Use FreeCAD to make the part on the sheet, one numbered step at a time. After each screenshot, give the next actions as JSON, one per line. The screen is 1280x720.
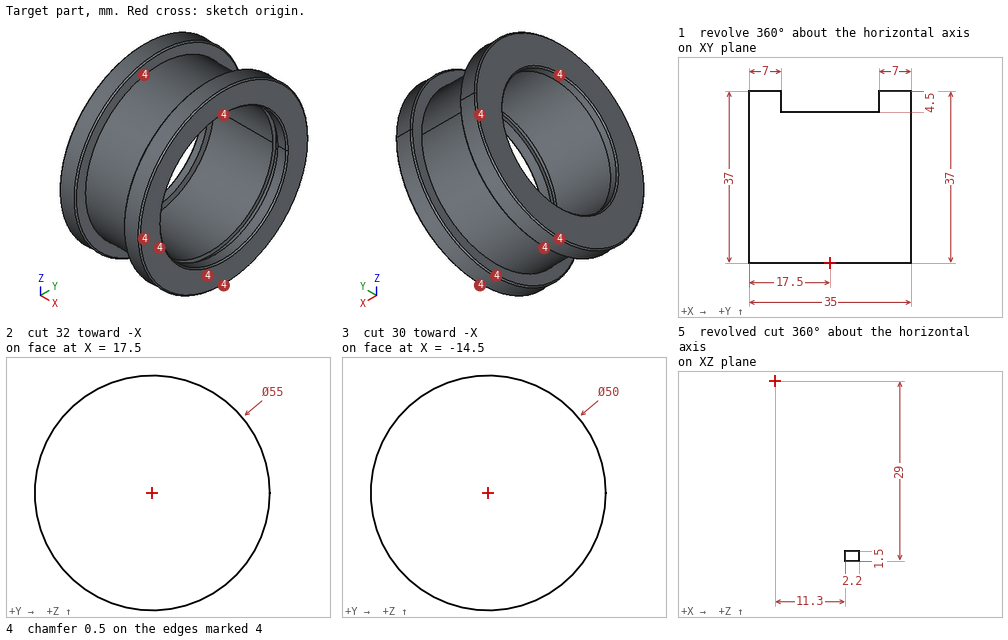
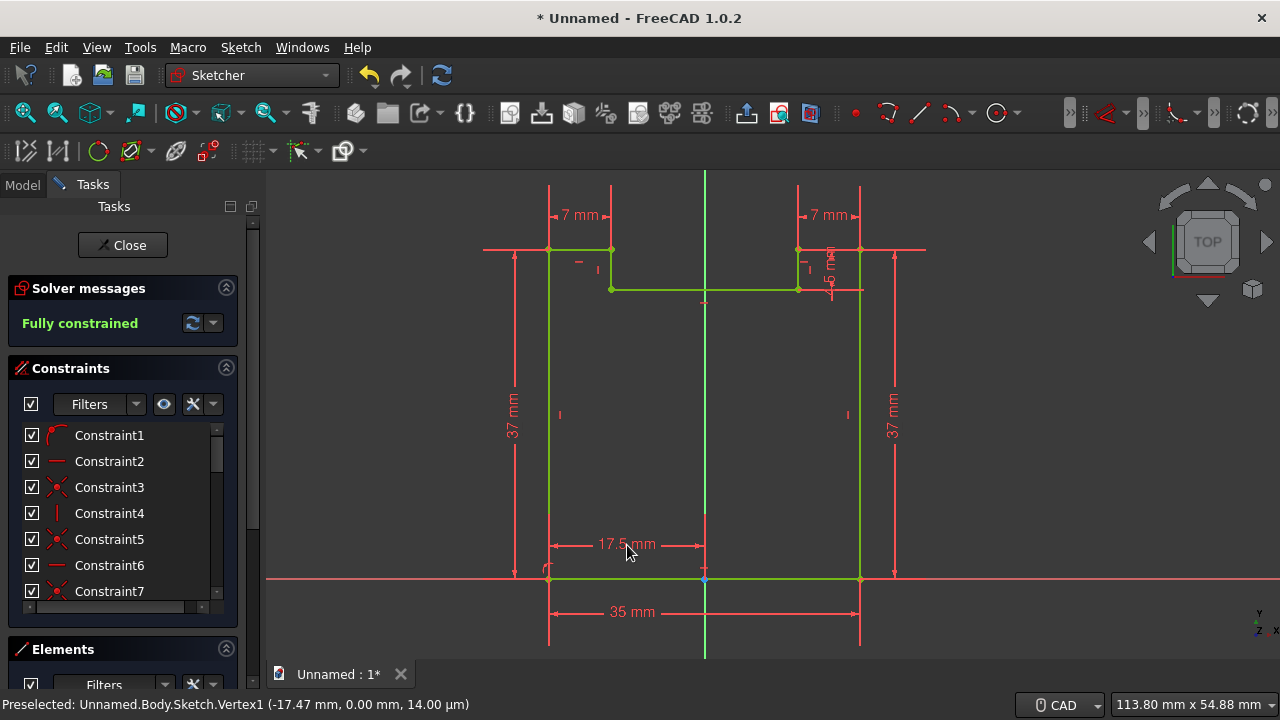
{"action": "left_click", "coordinate": [123, 245]}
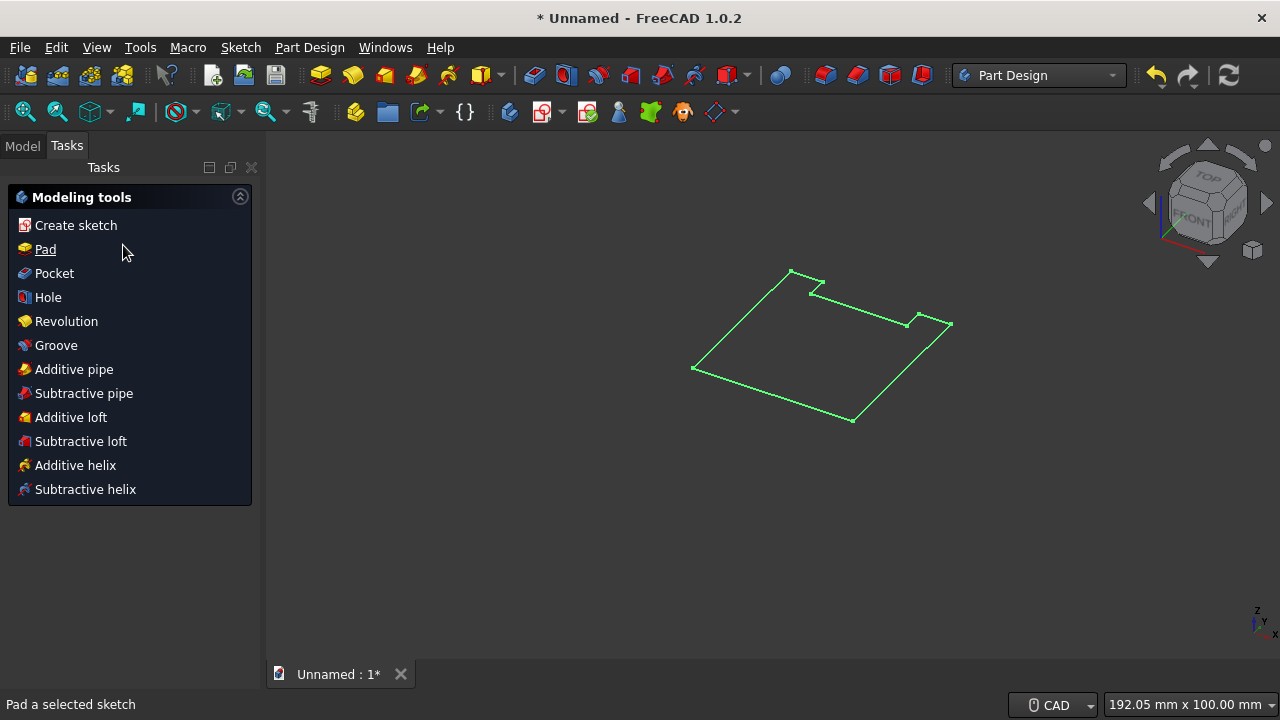
{"action": "left_click", "coordinate": [354, 76]}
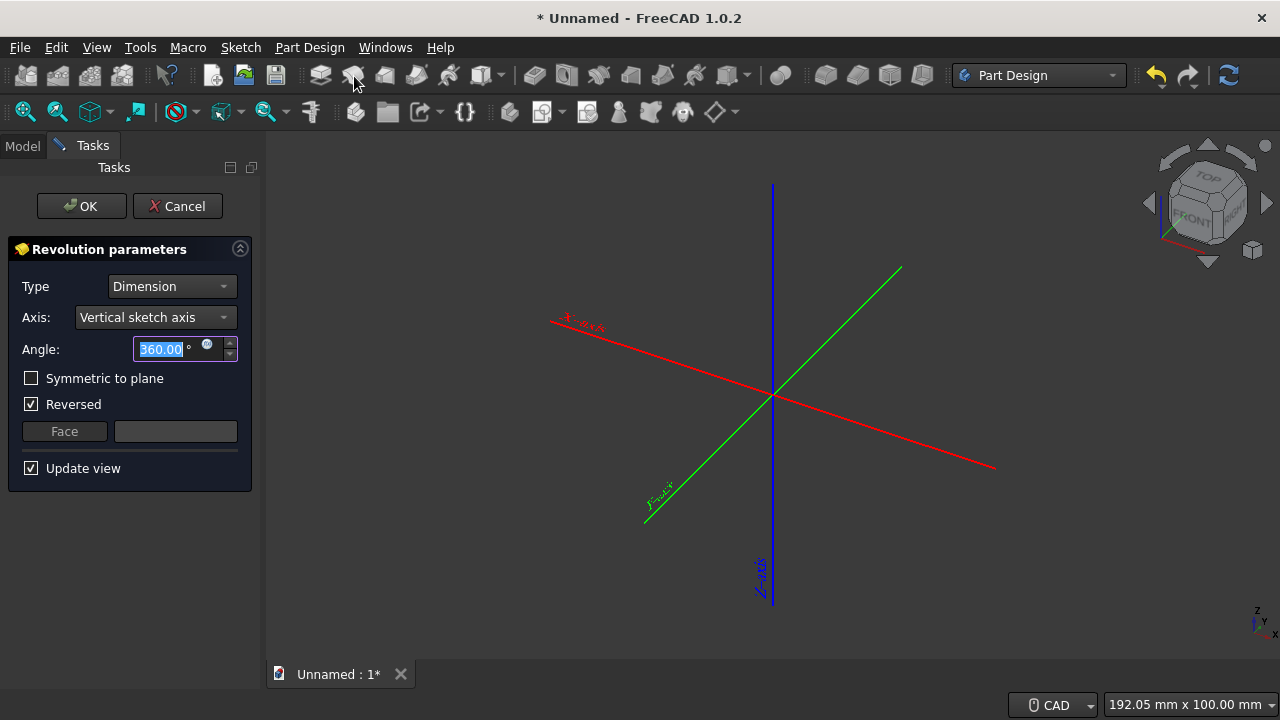
{"action": "left_click", "coordinate": [156, 318]}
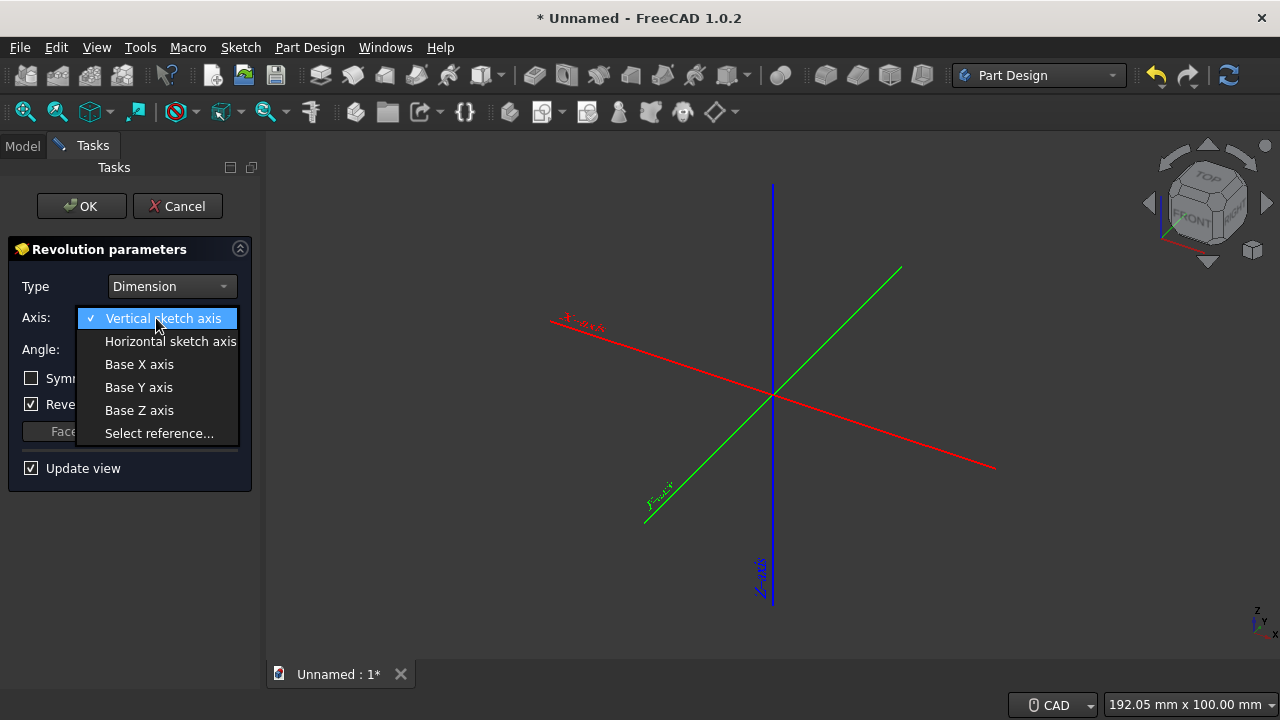
{"action": "left_click", "coordinate": [156, 342]}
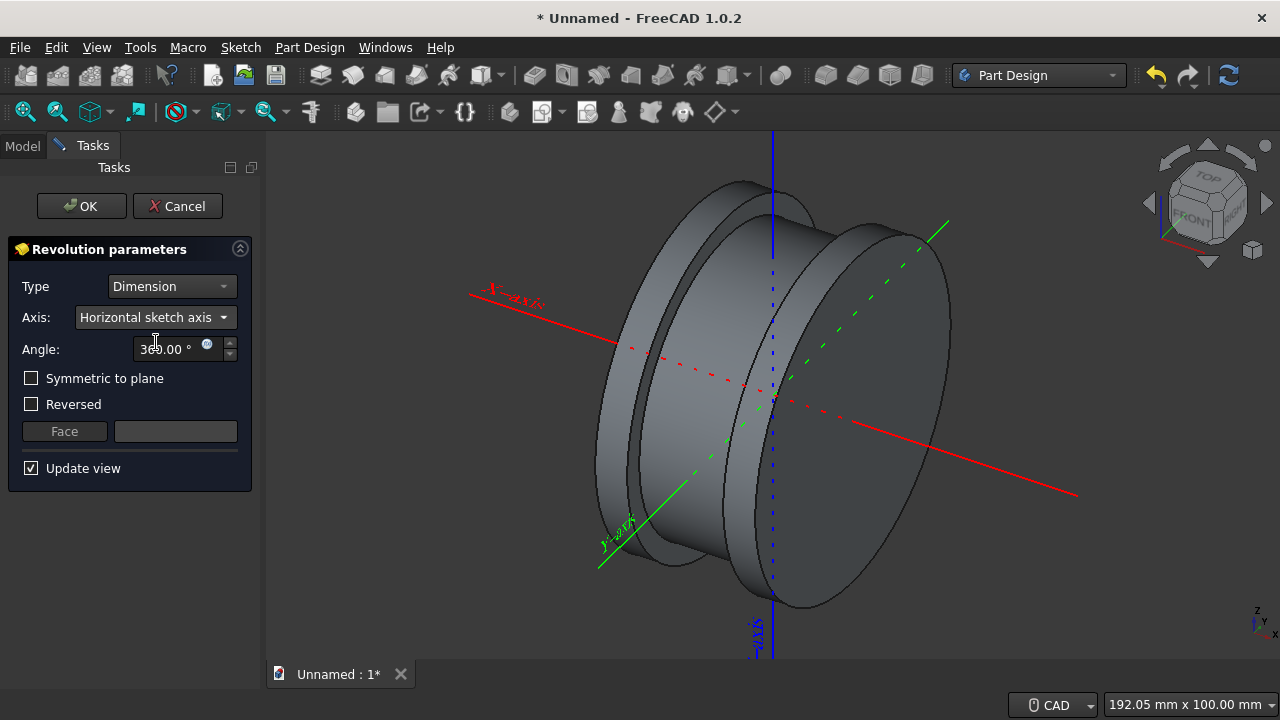
{"action": "left_click", "coordinate": [82, 206]}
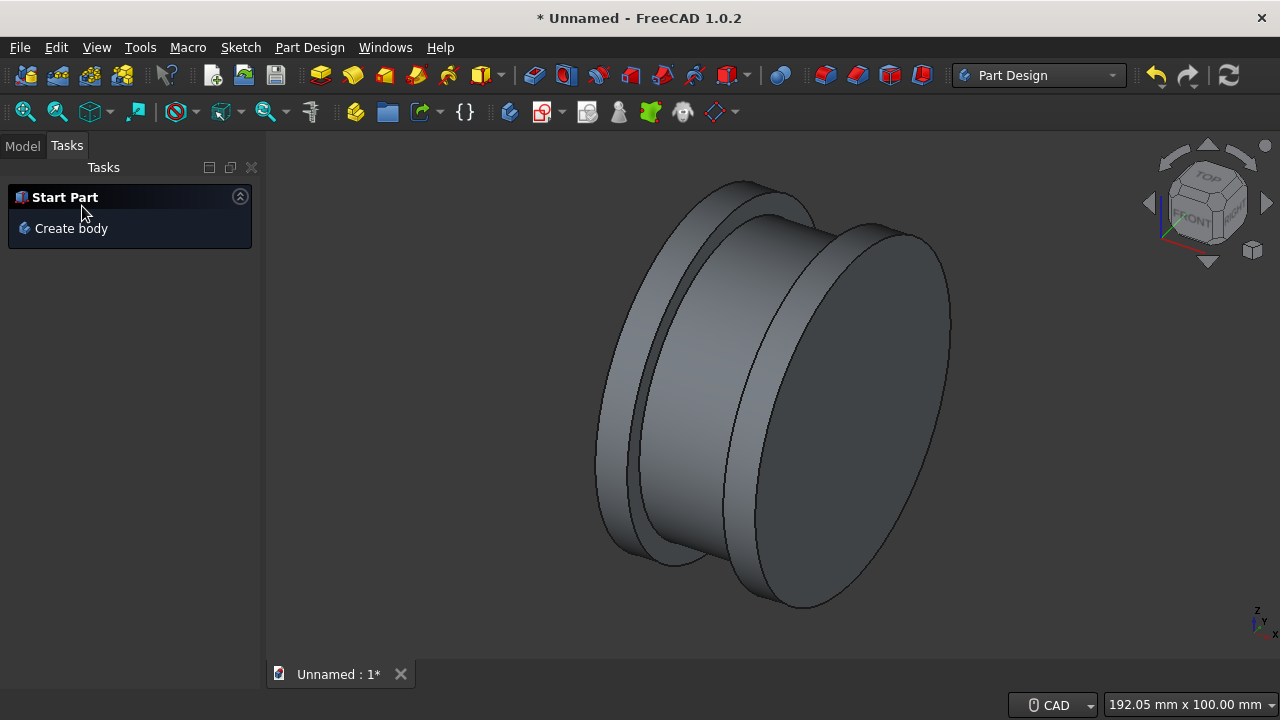
{"action": "key", "text": "v f"}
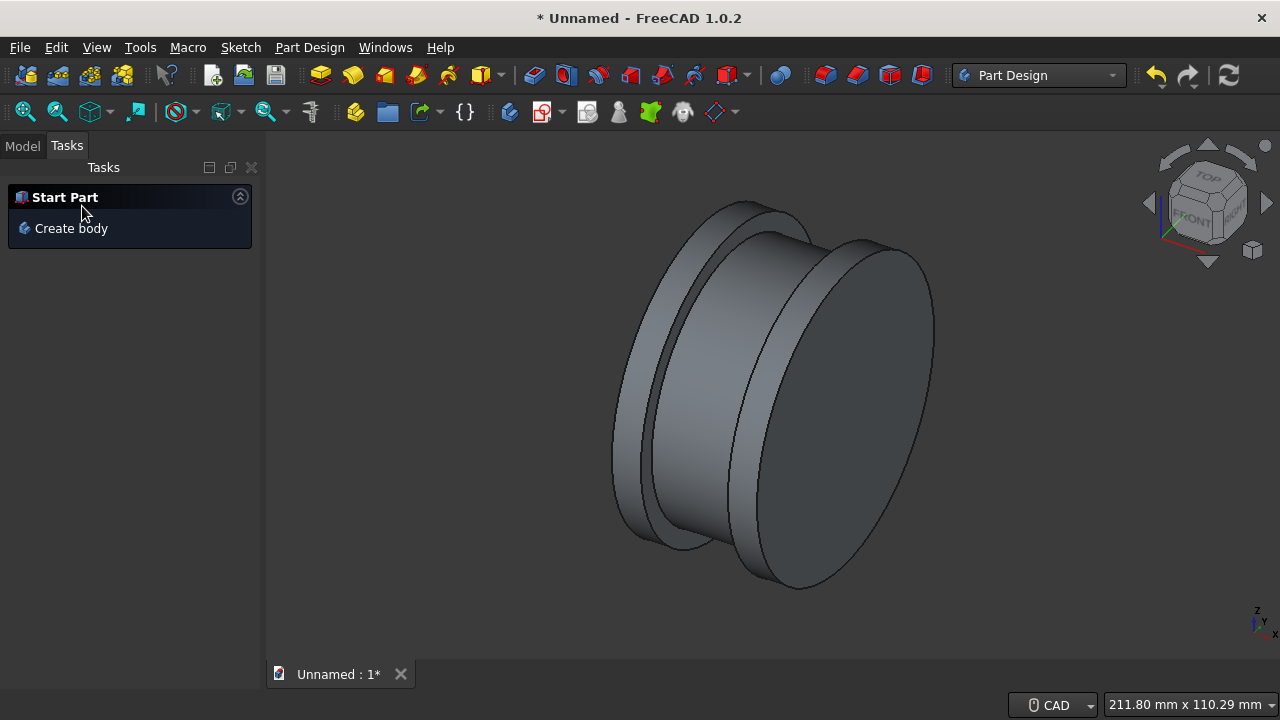
{"action": "left_click", "coordinate": [845, 418]}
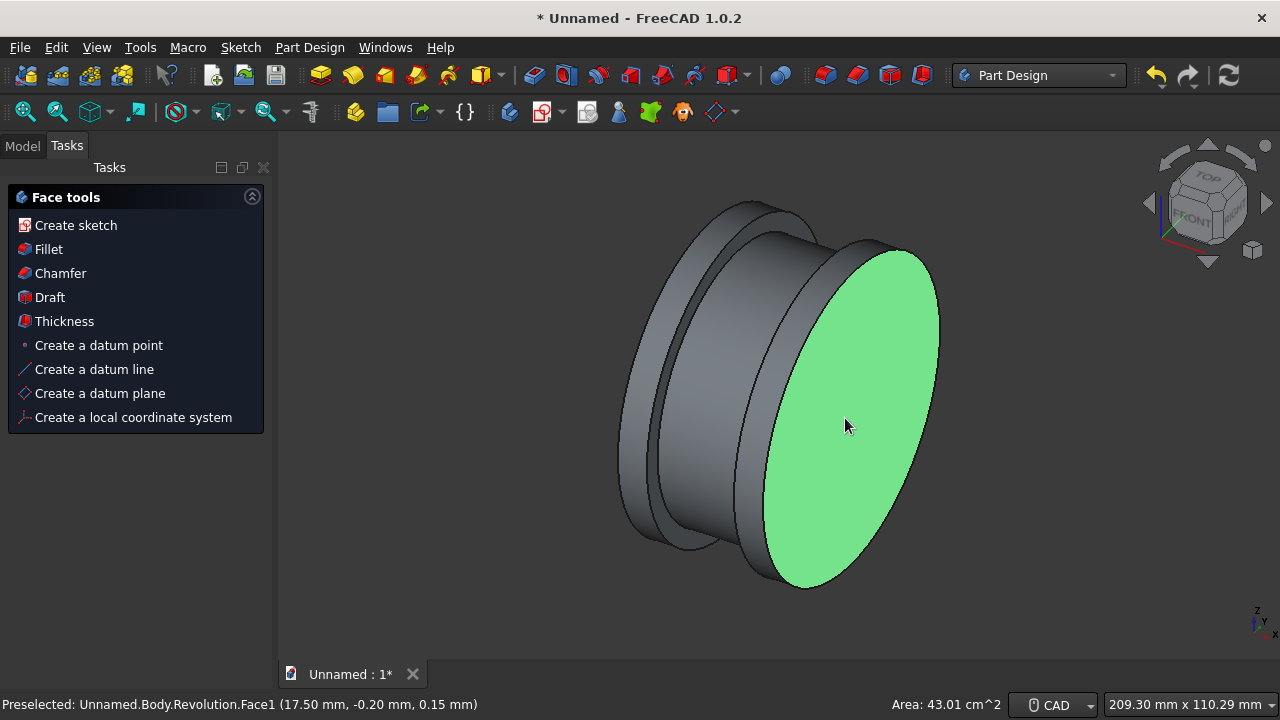
{"action": "left_click", "coordinate": [542, 112]}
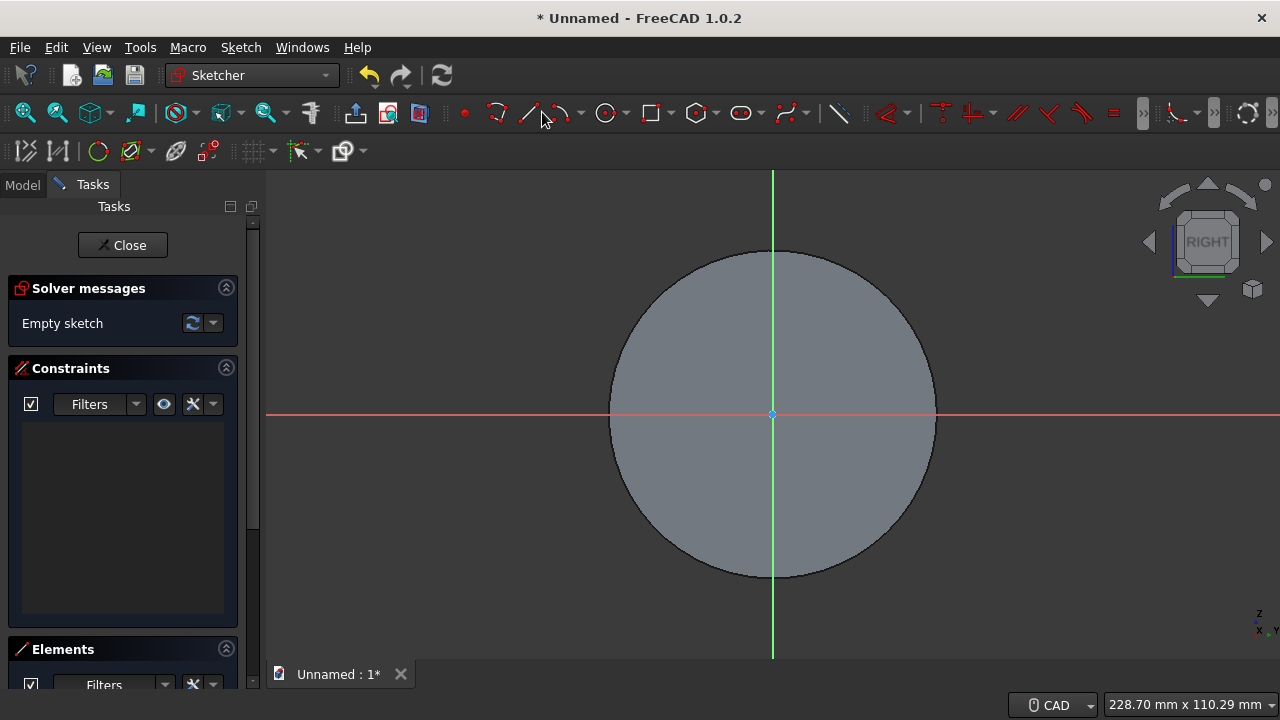
{"action": "left_click", "coordinate": [606, 114]}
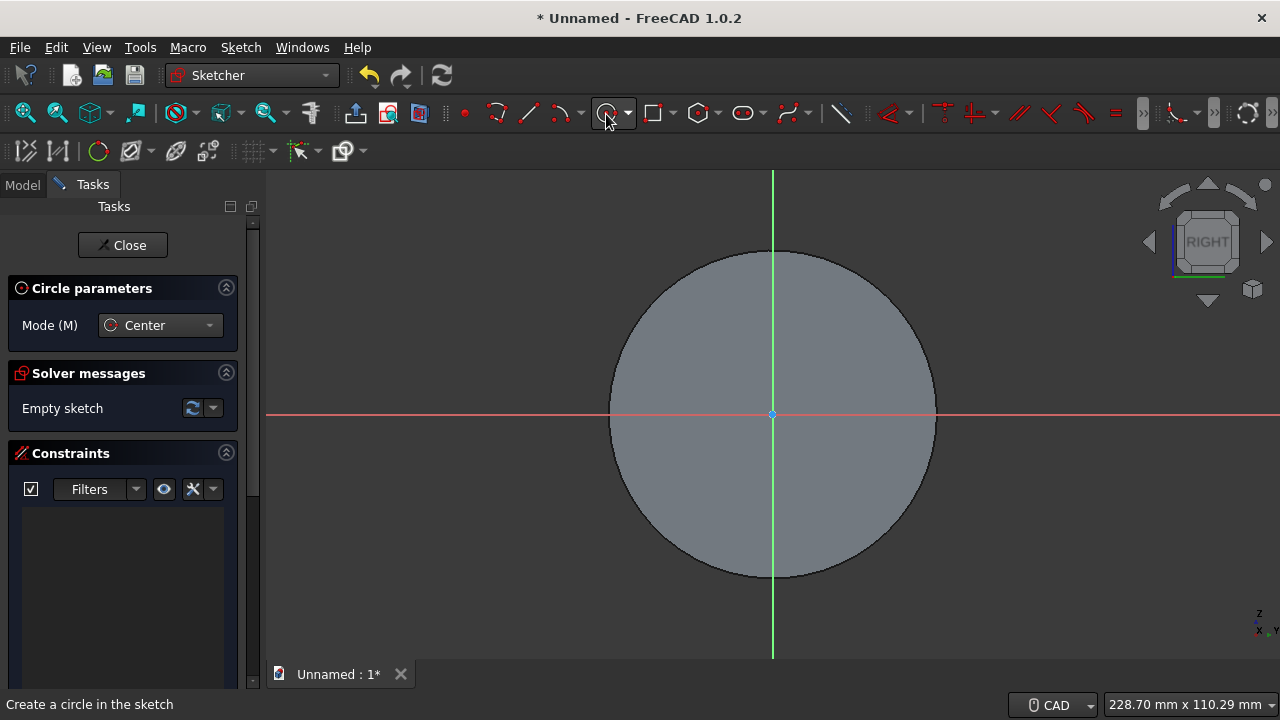
{"action": "left_click", "coordinate": [773, 414]}
{"action": "left_click", "coordinate": [859, 328]}
{"action": "key", "text": "Escape"}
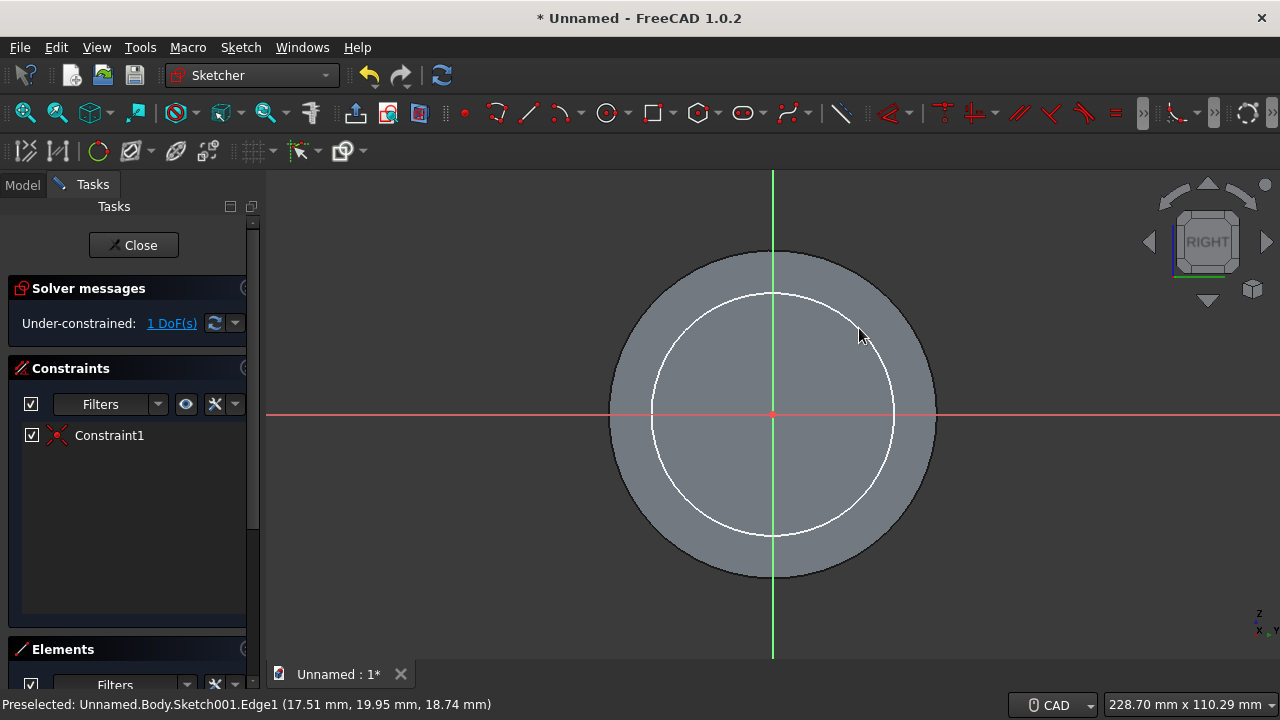
{"action": "left_click", "coordinate": [888, 114]}